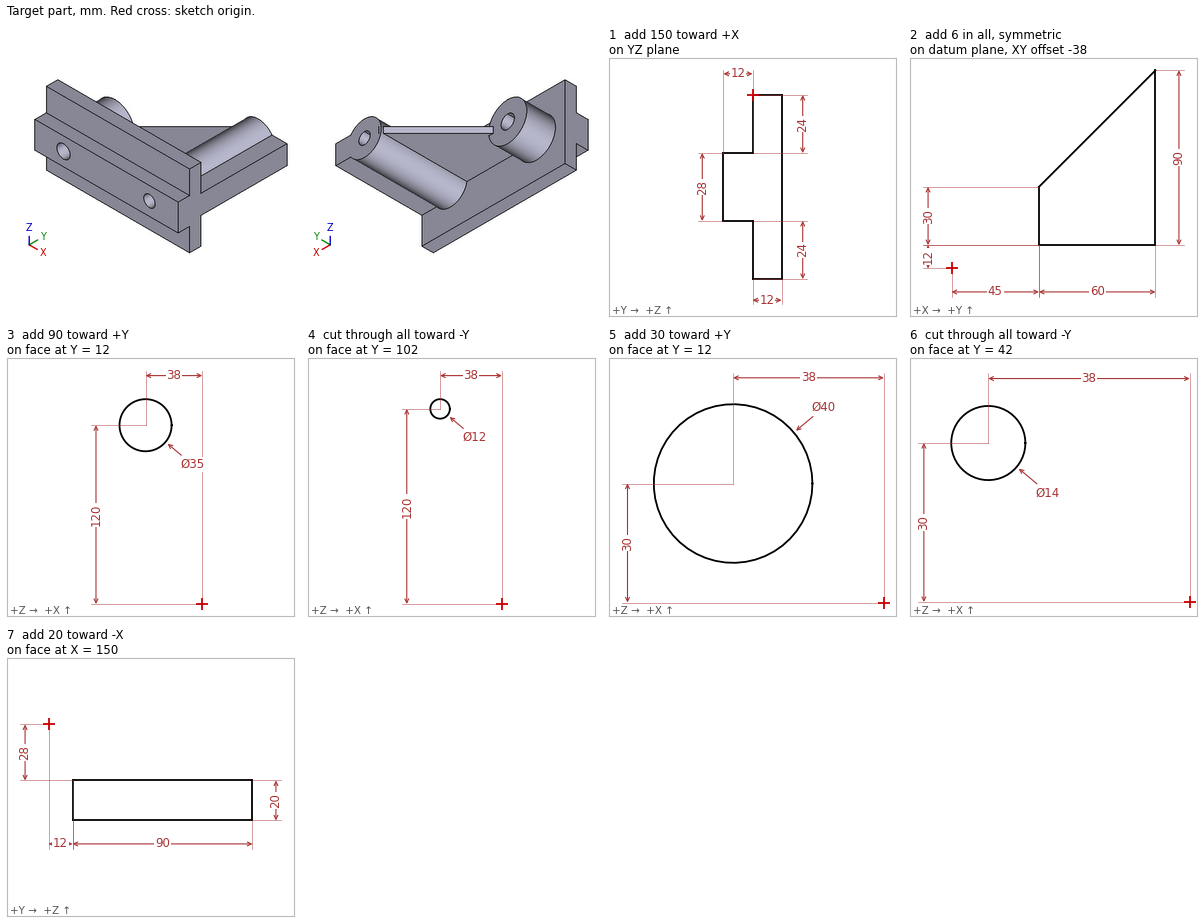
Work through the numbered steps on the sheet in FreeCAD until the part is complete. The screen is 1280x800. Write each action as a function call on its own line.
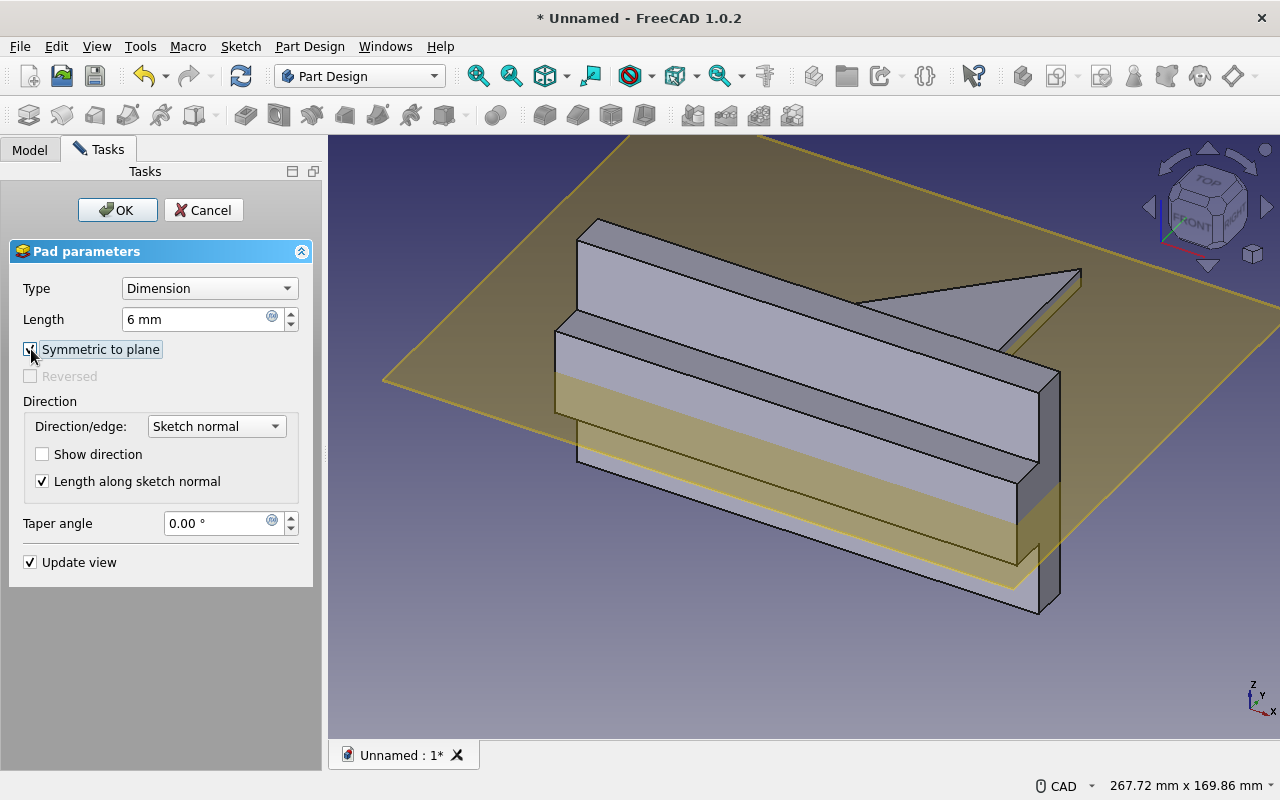
click(118, 210)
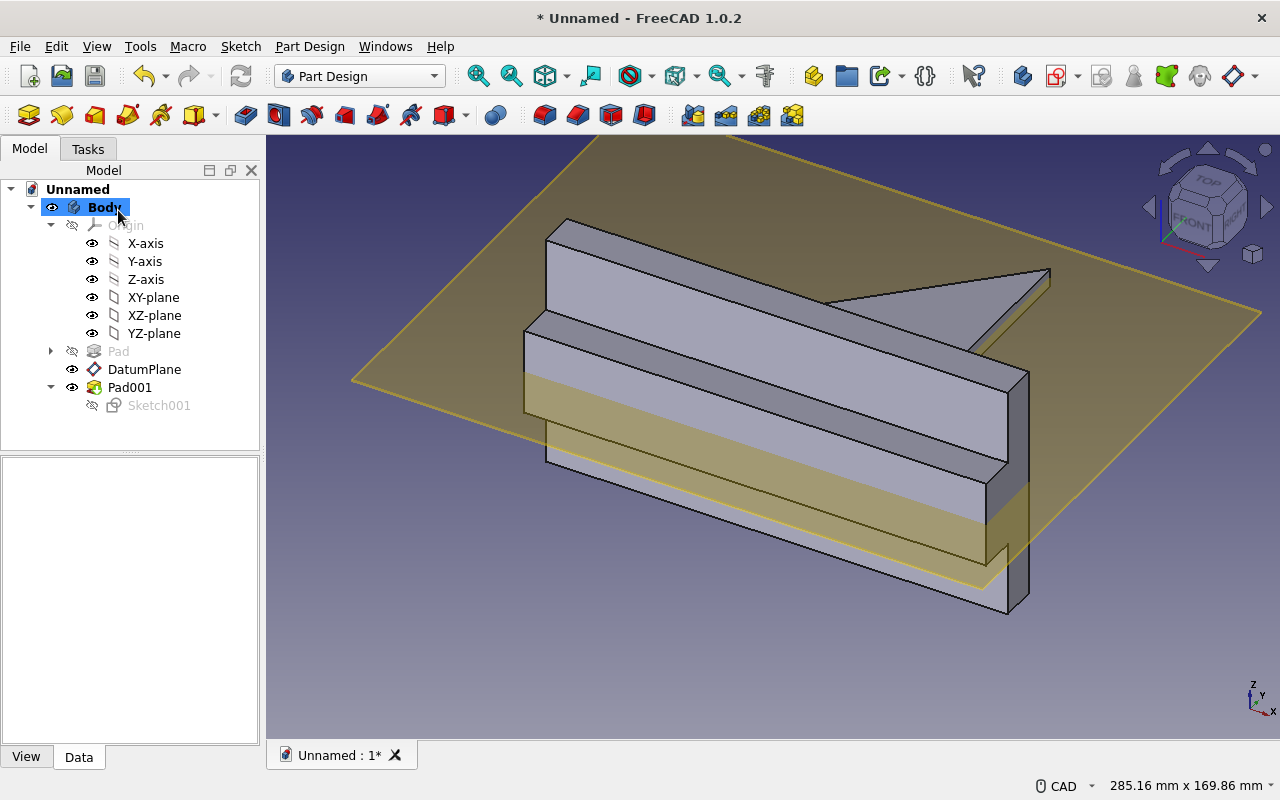
click(117, 369)
key(space)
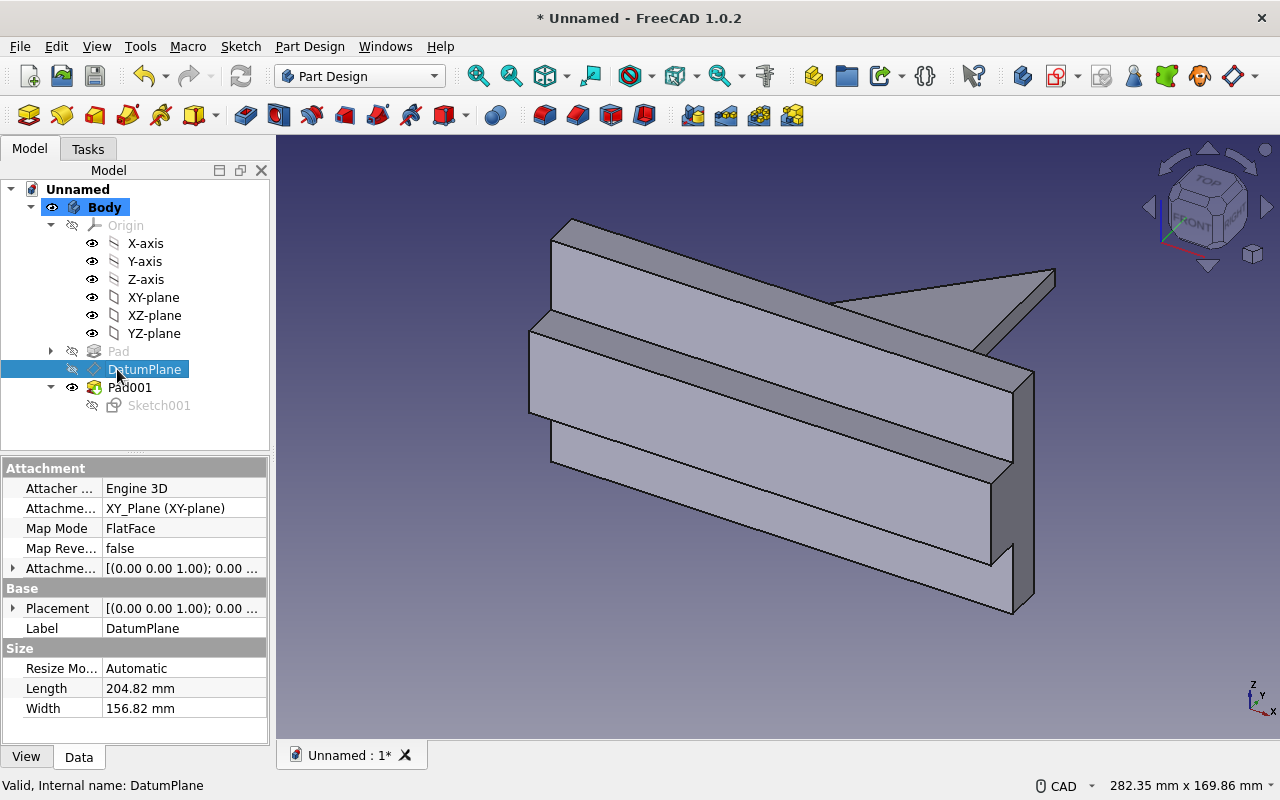
click(479, 76)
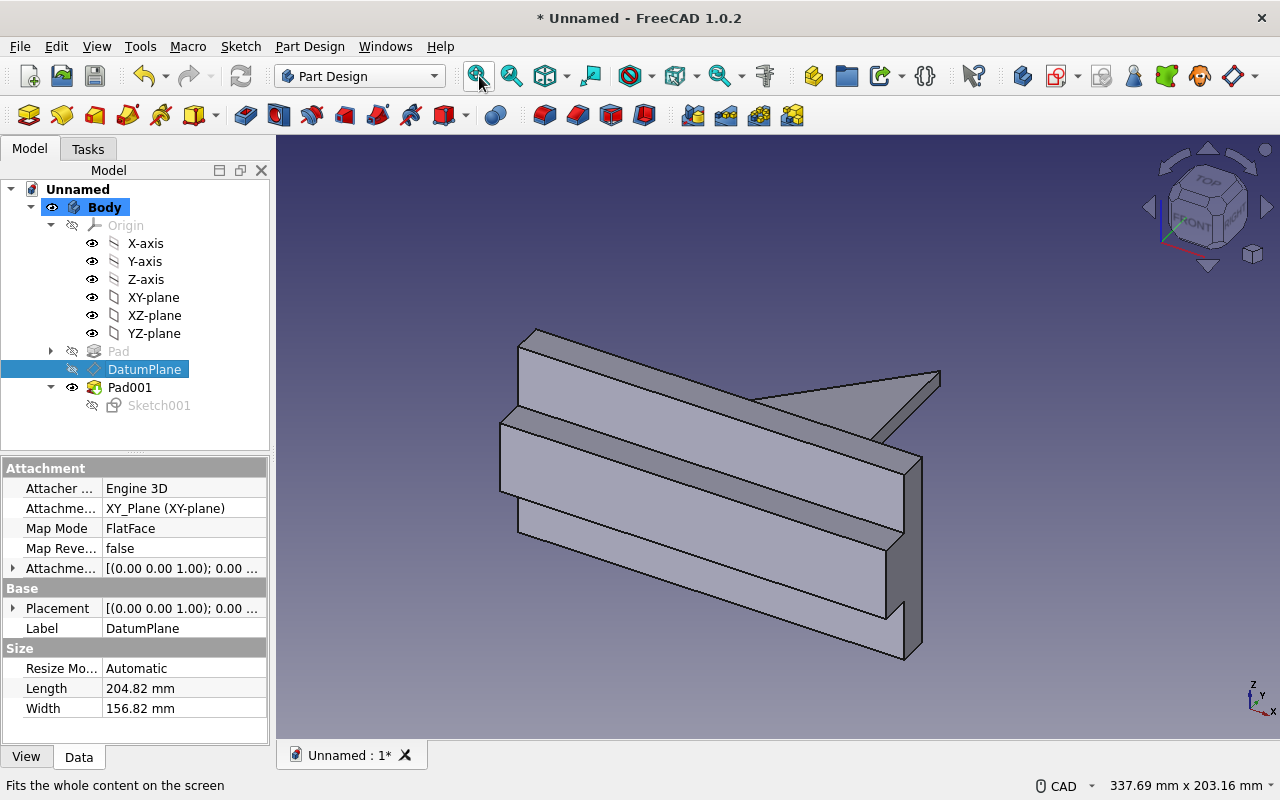
key(4)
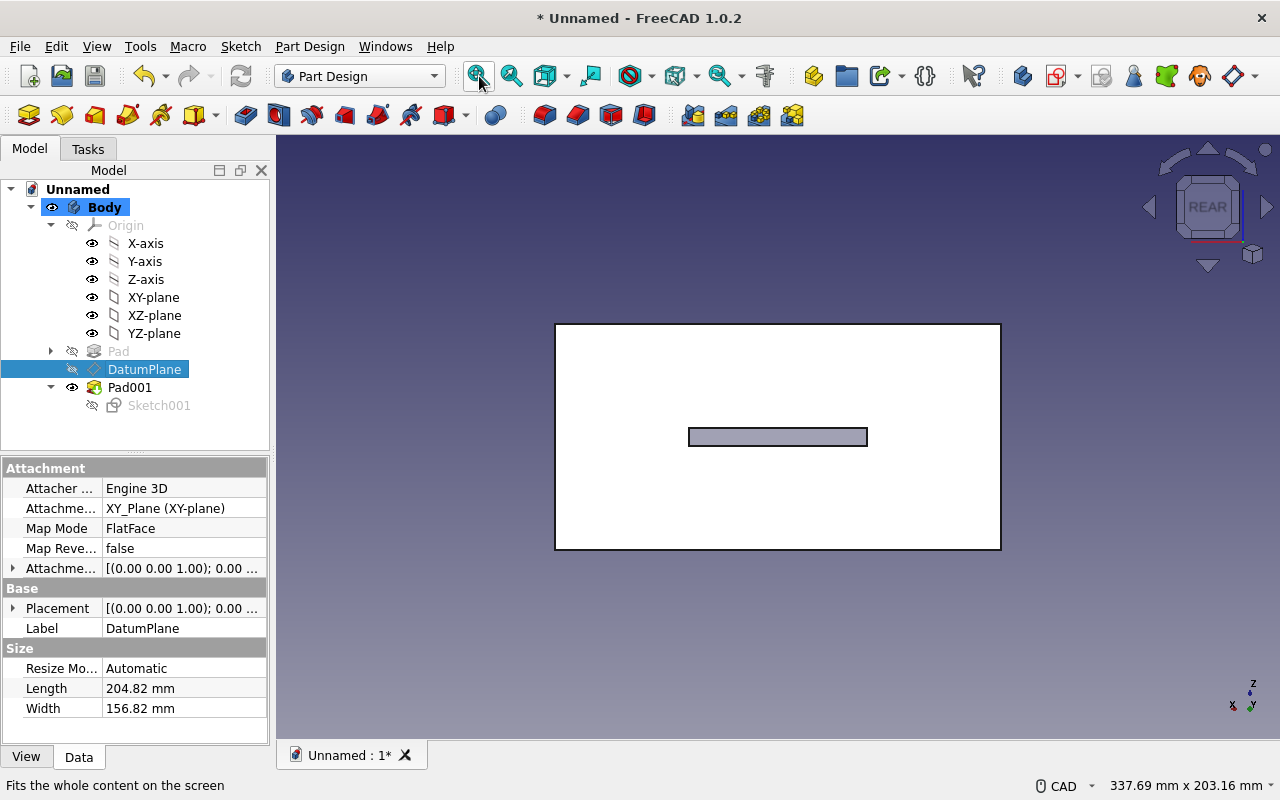
click(479, 76)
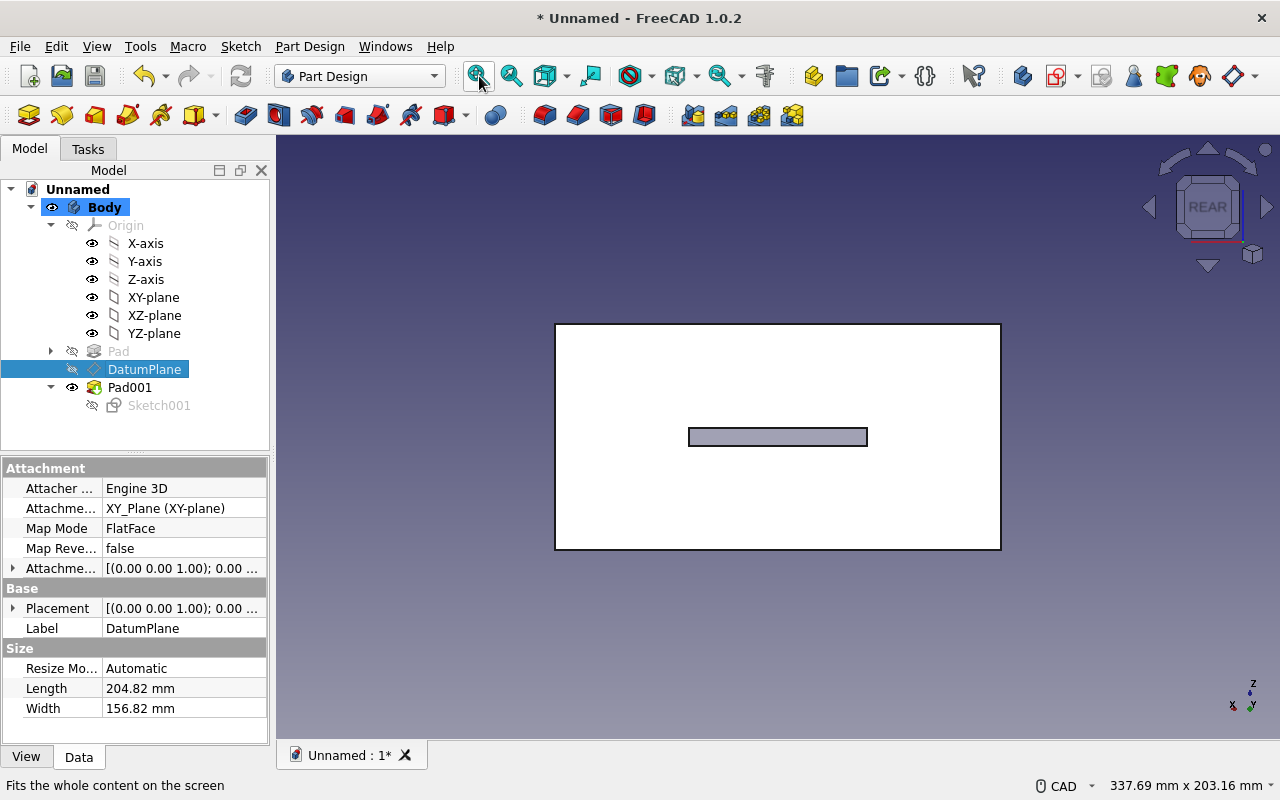
click(905, 371)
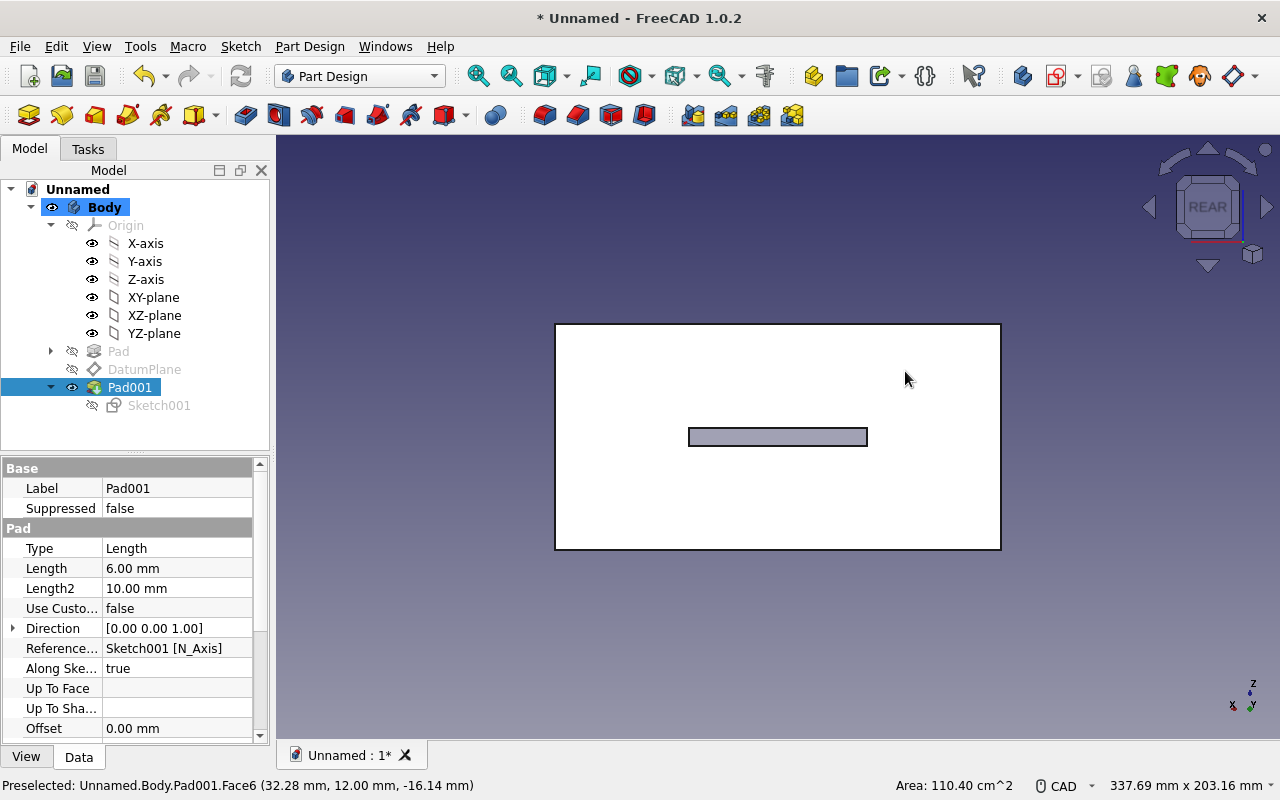
click(1056, 76)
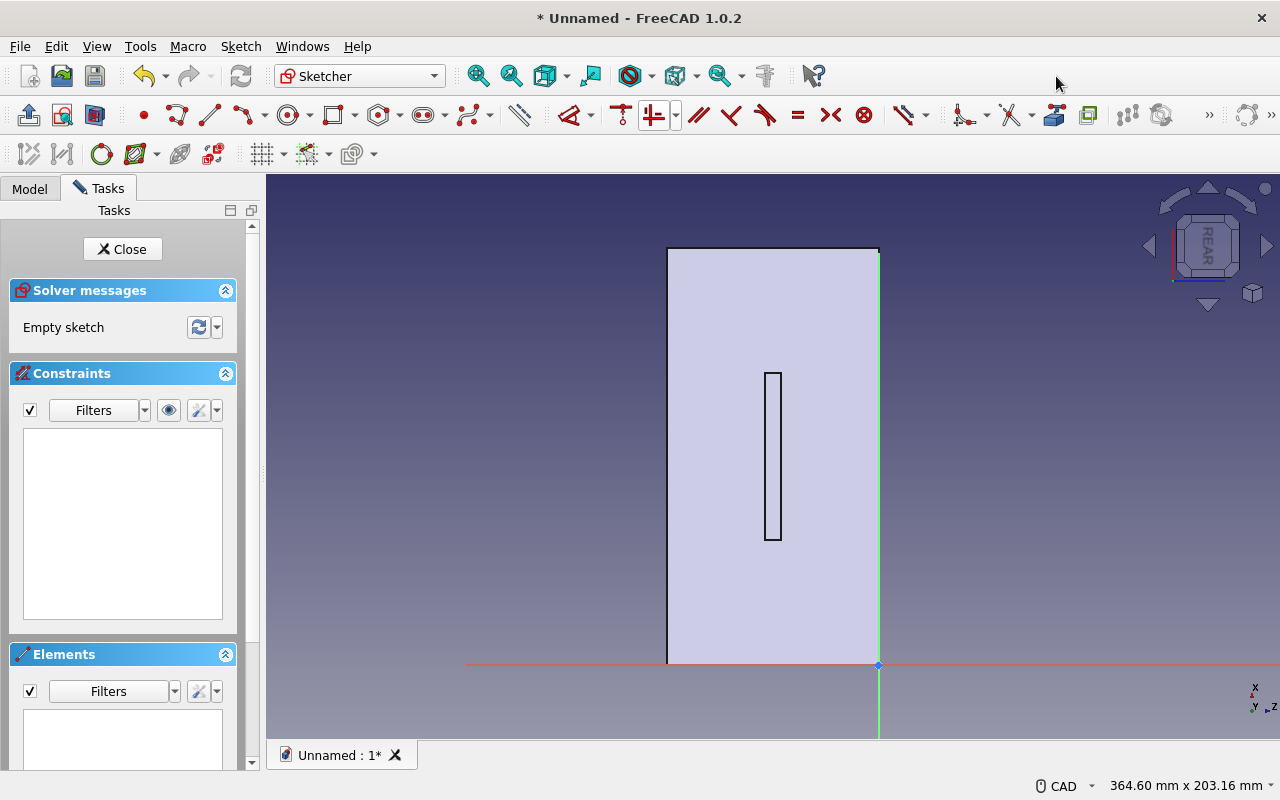
scroll(795, 290, up, 7)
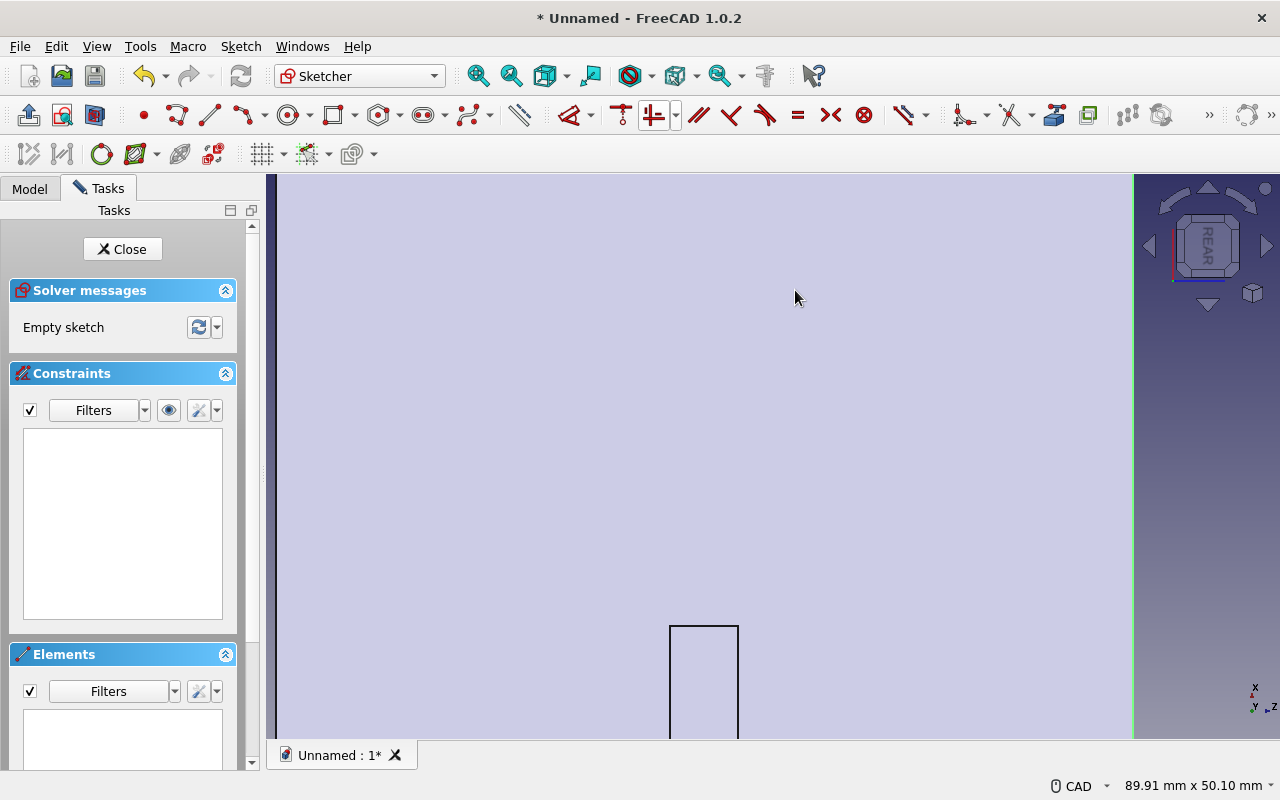
click(288, 116)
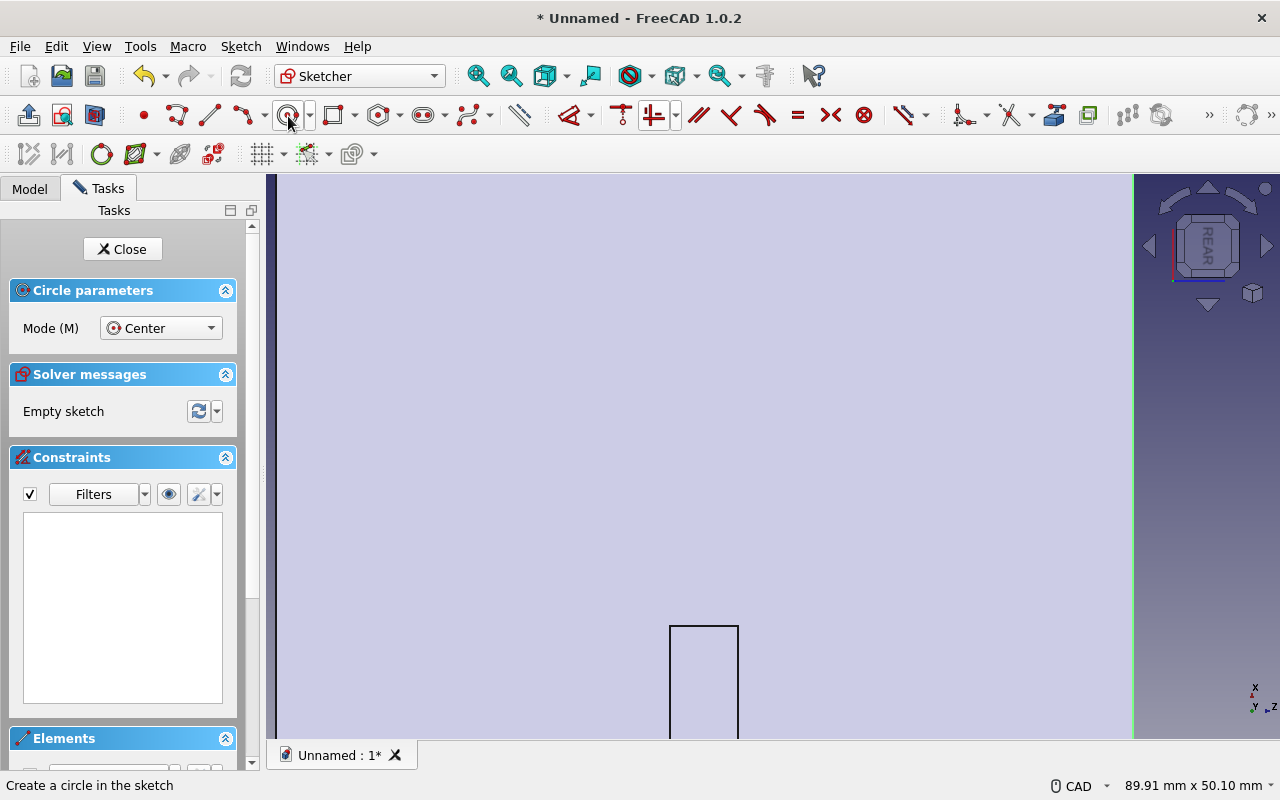
click(704, 457)
move(844, 317)